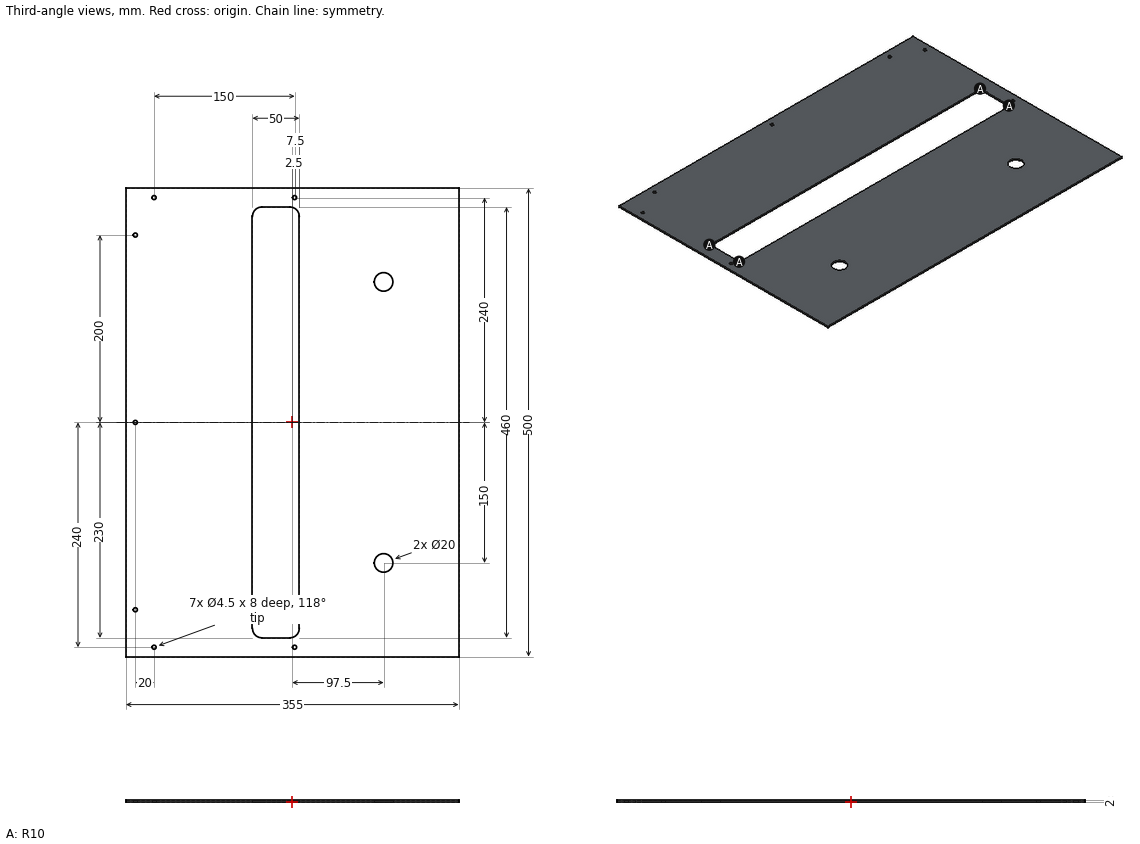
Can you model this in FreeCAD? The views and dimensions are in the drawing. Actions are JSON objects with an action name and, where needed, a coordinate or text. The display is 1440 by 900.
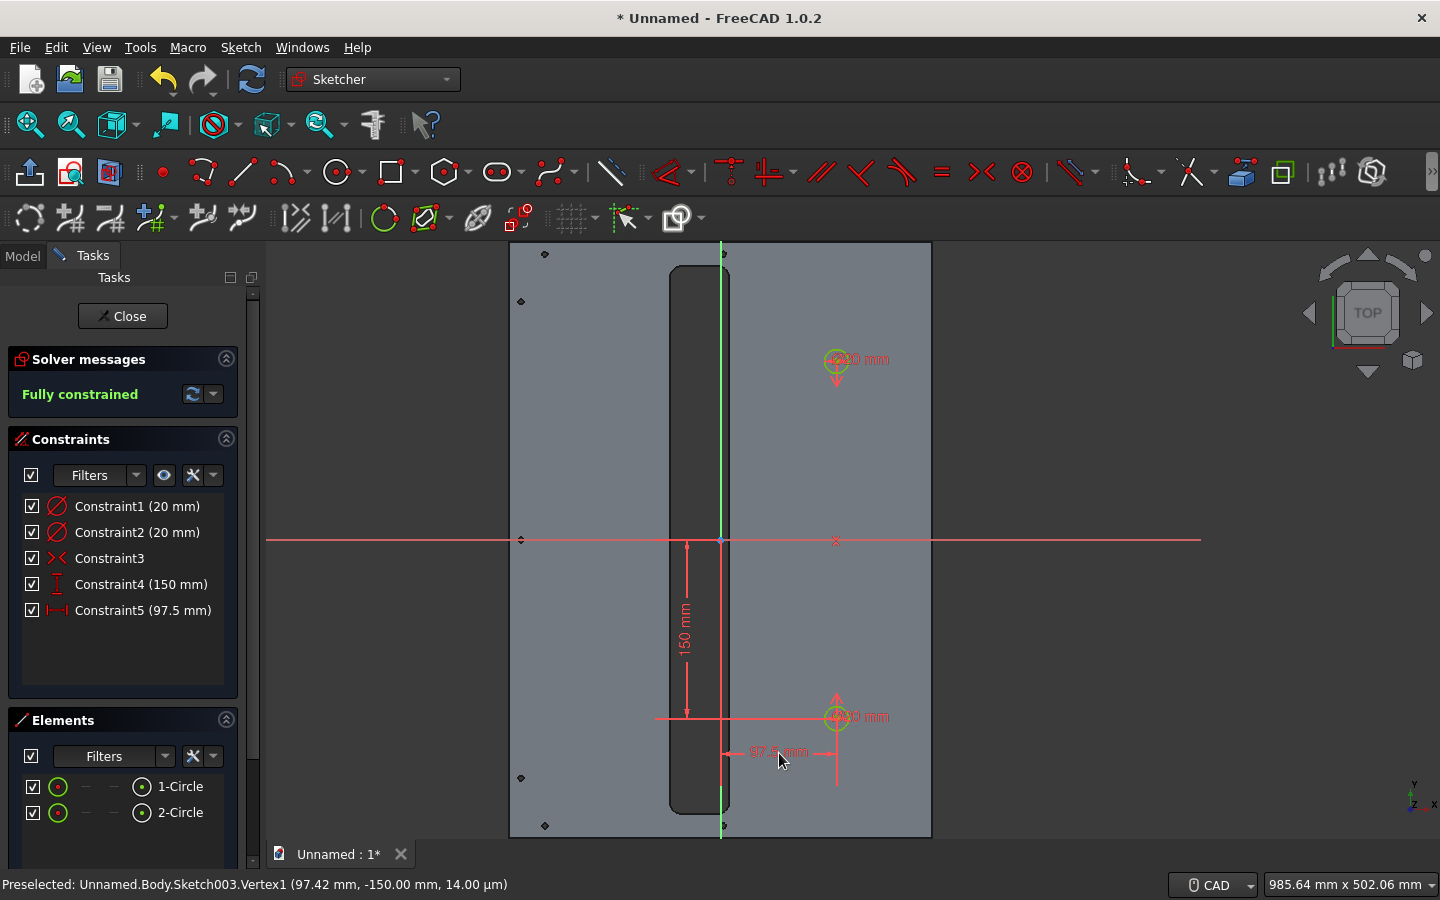
{"action": "left_click", "coordinate": [123, 316]}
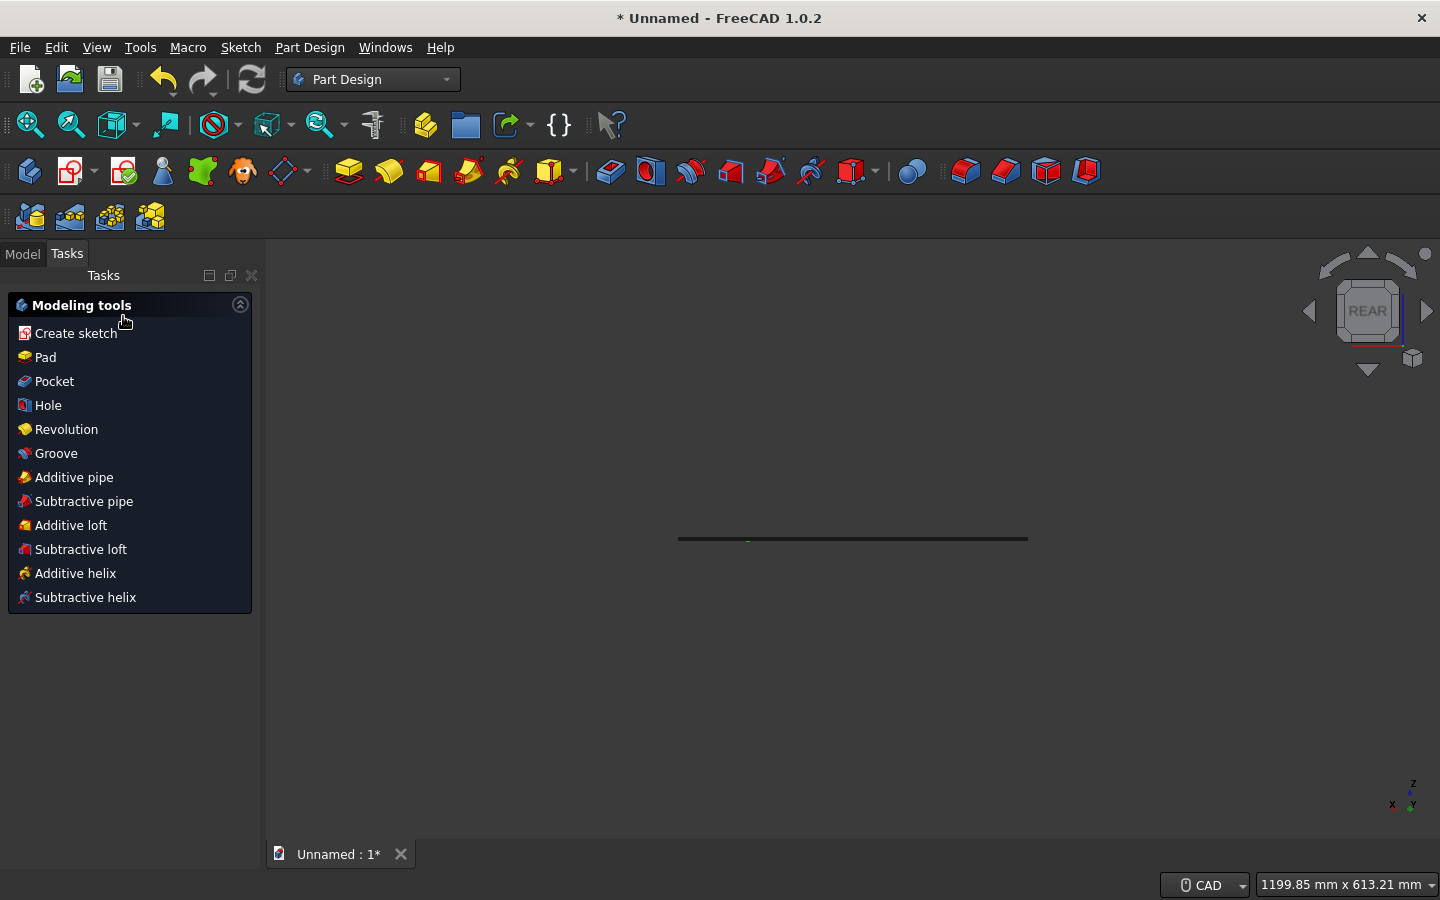
{"action": "left_click", "coordinate": [612, 172]}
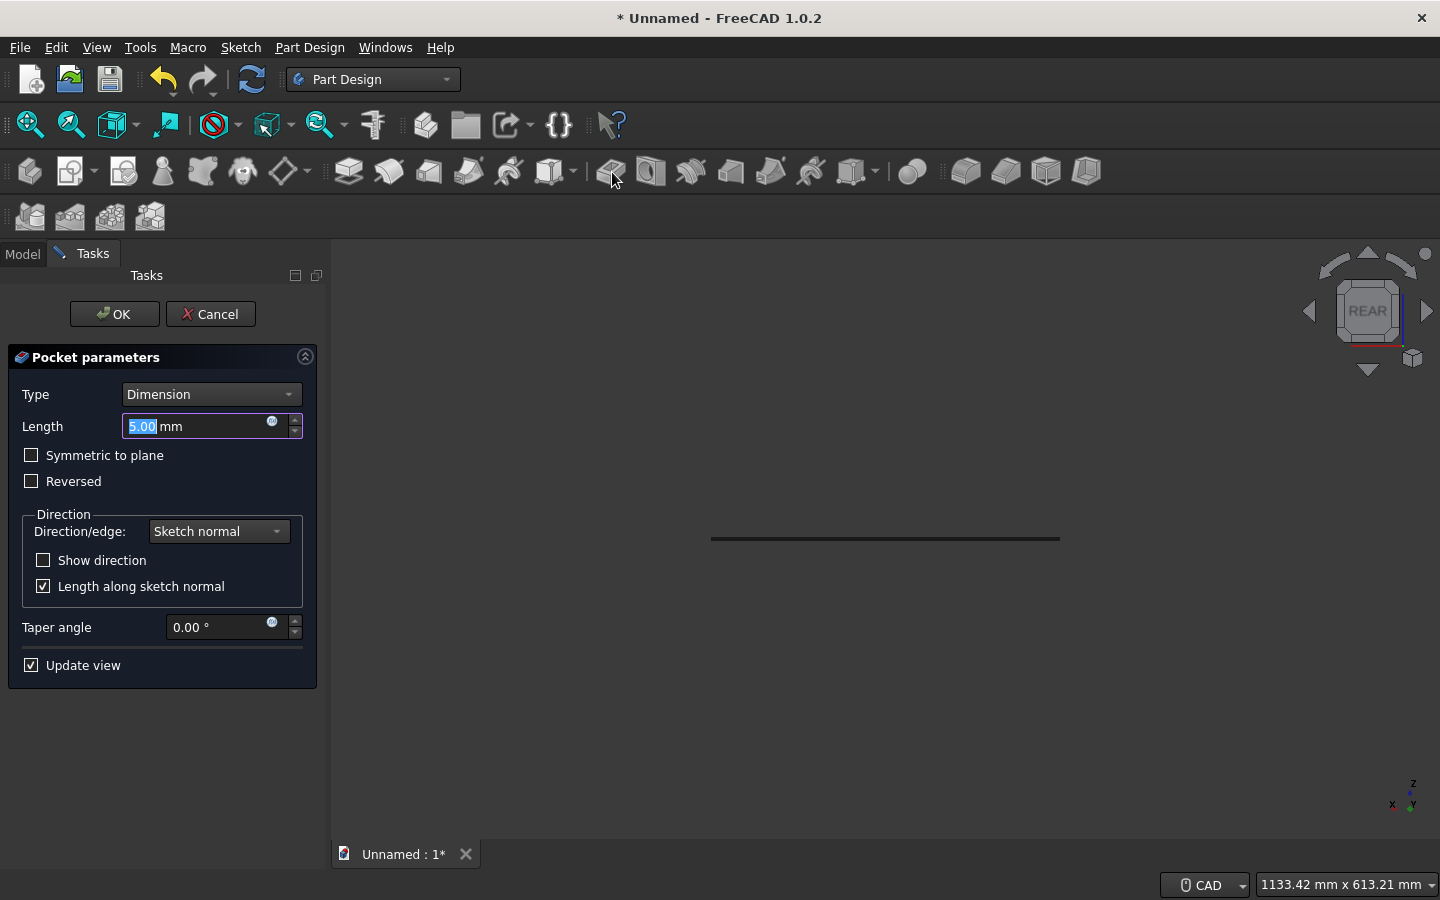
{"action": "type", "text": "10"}
{"action": "key", "text": "Tab"}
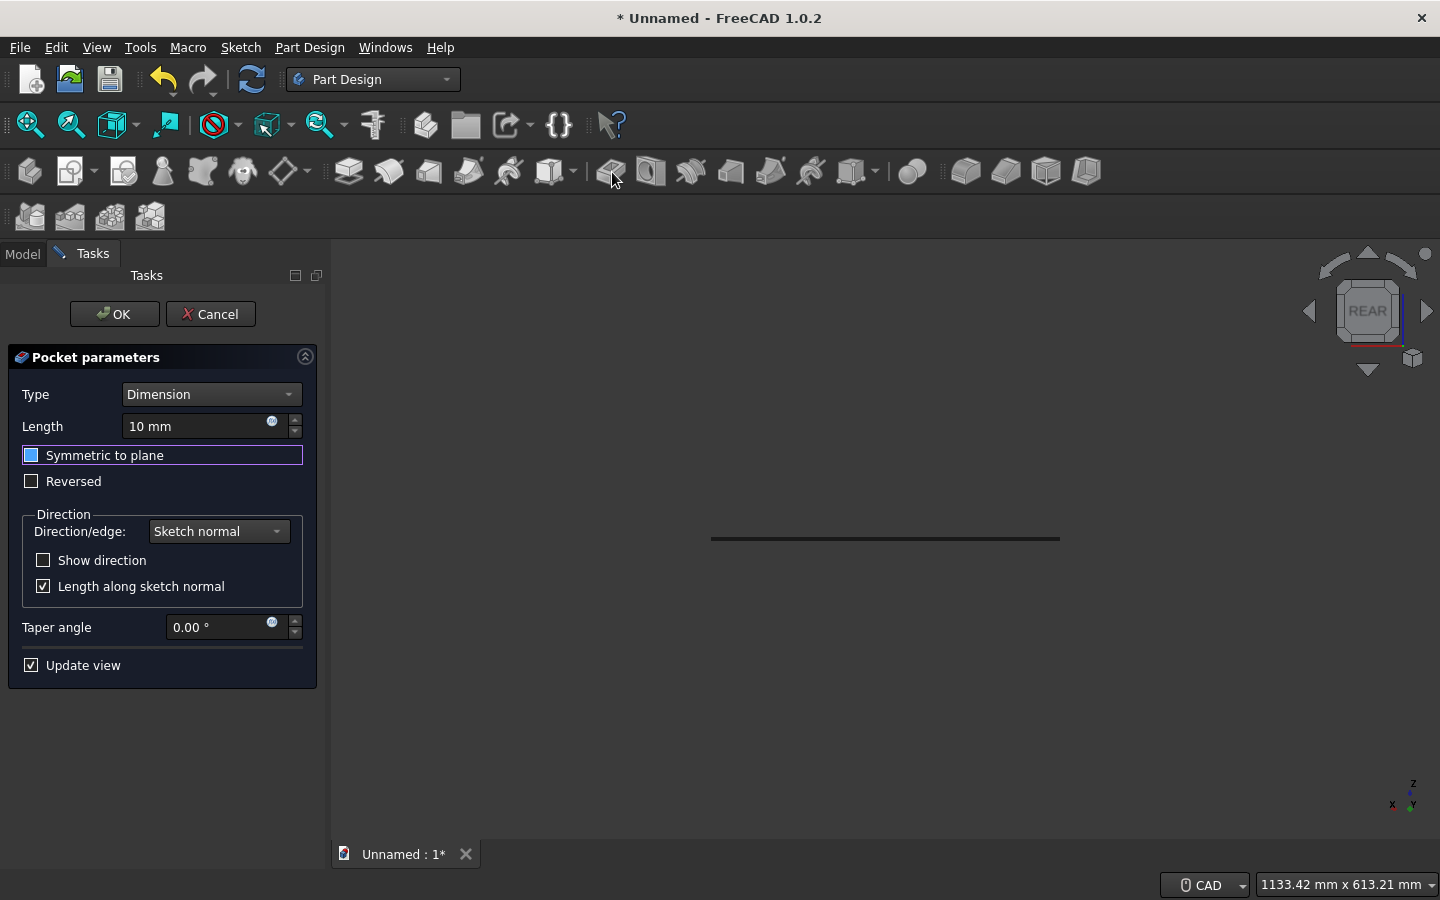
{"action": "left_click", "coordinate": [30, 481]}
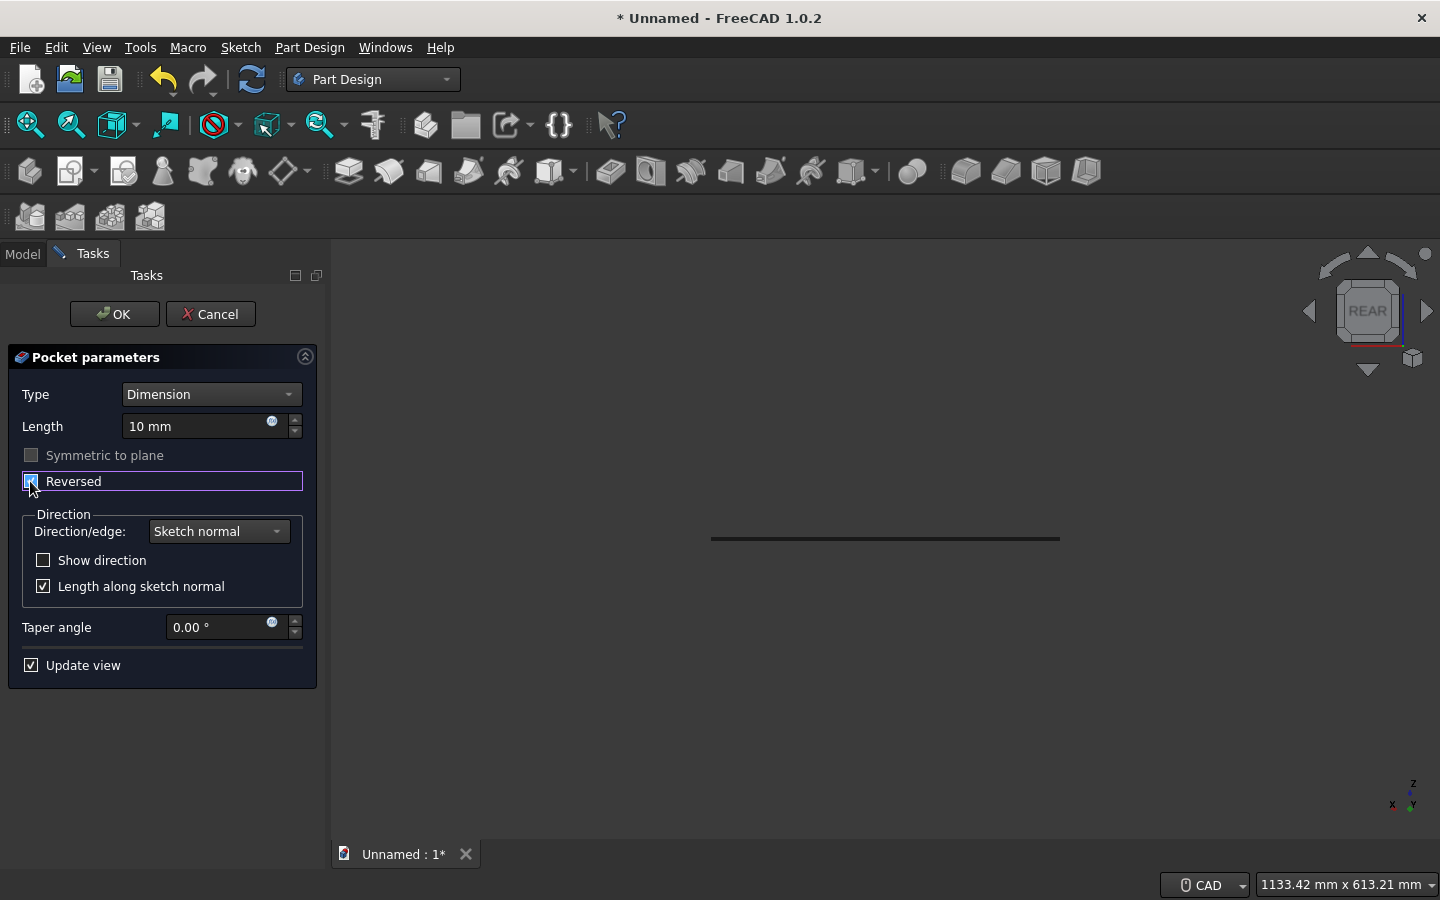
{"action": "left_click", "coordinate": [115, 314]}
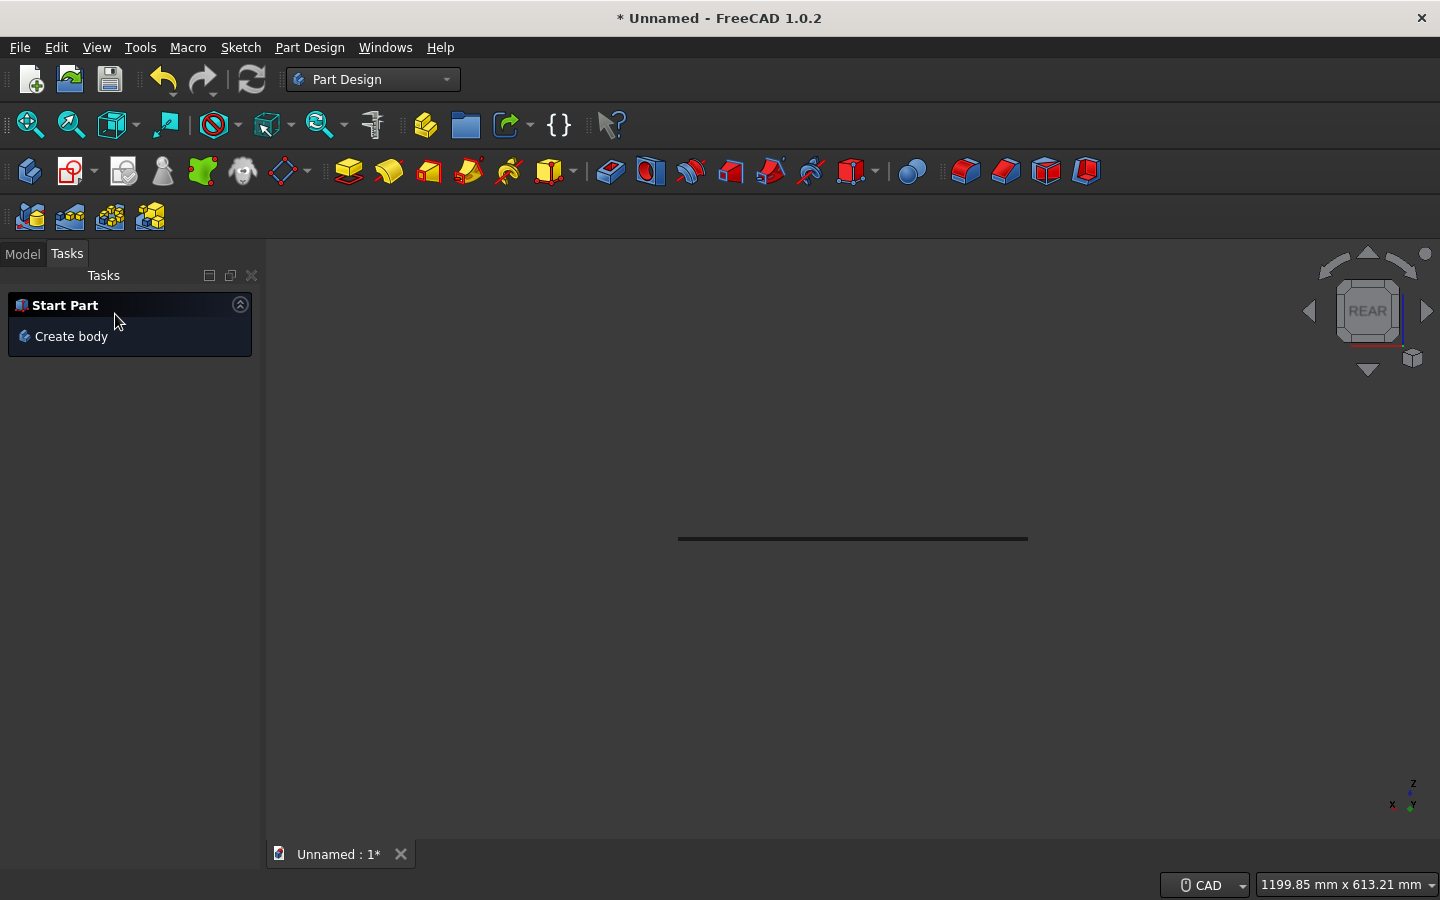
{"action": "key", "text": "0"}